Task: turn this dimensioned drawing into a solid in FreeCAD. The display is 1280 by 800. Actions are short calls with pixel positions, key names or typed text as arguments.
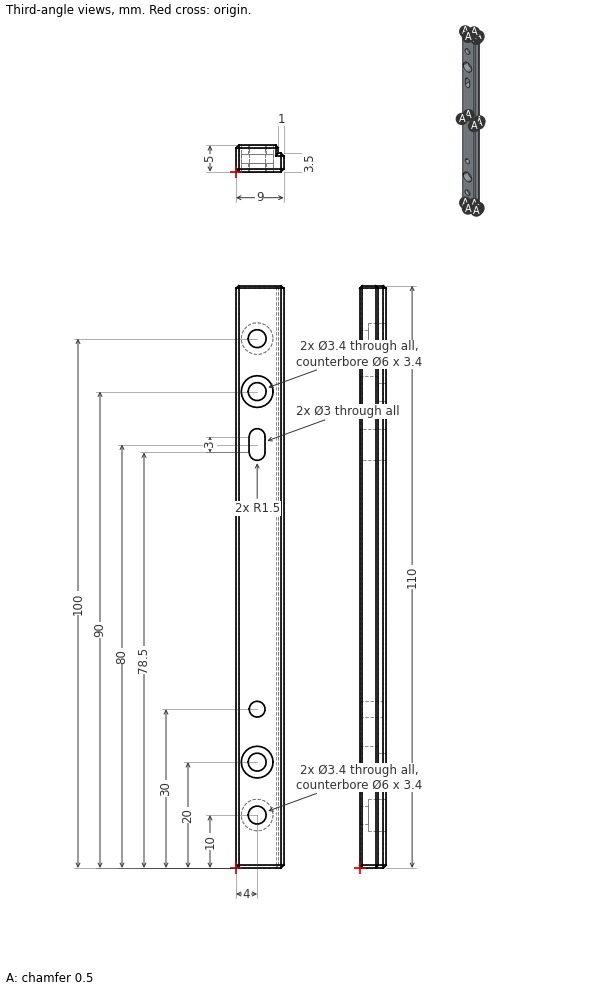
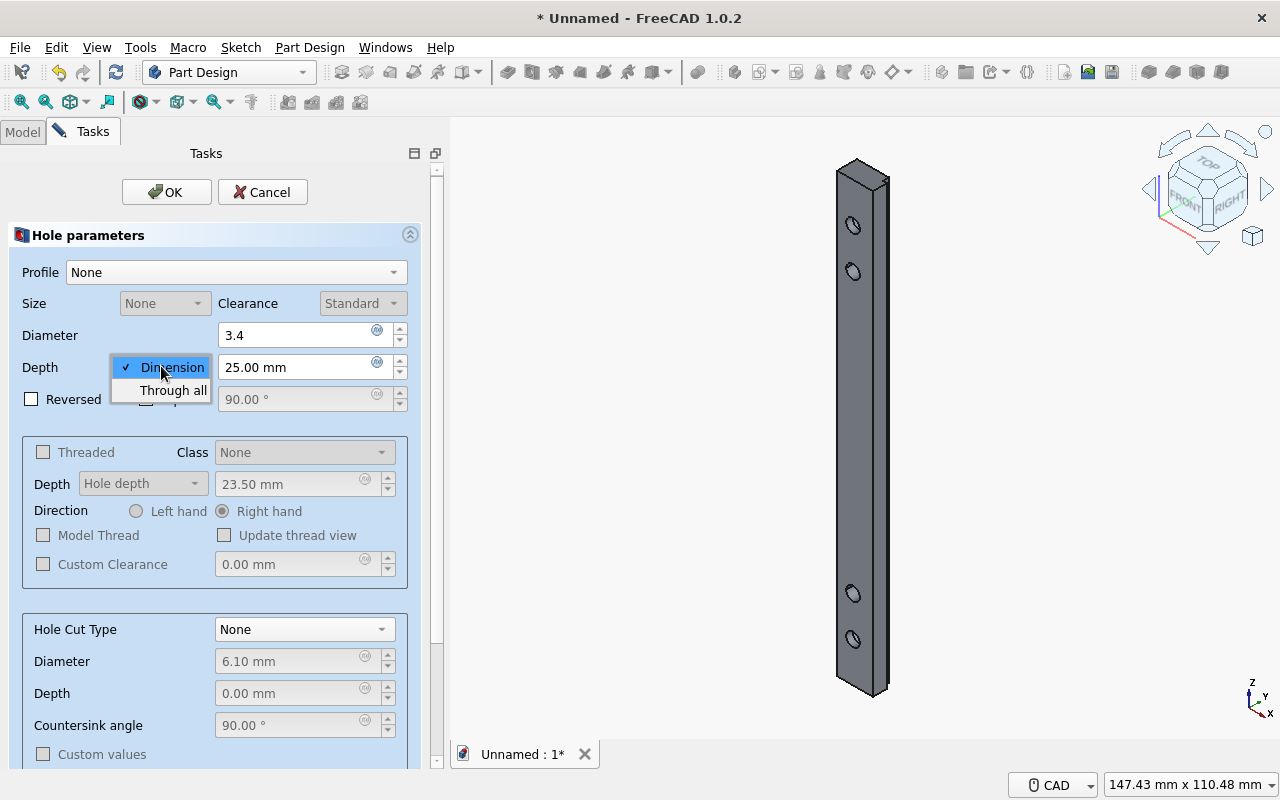
click(160, 390)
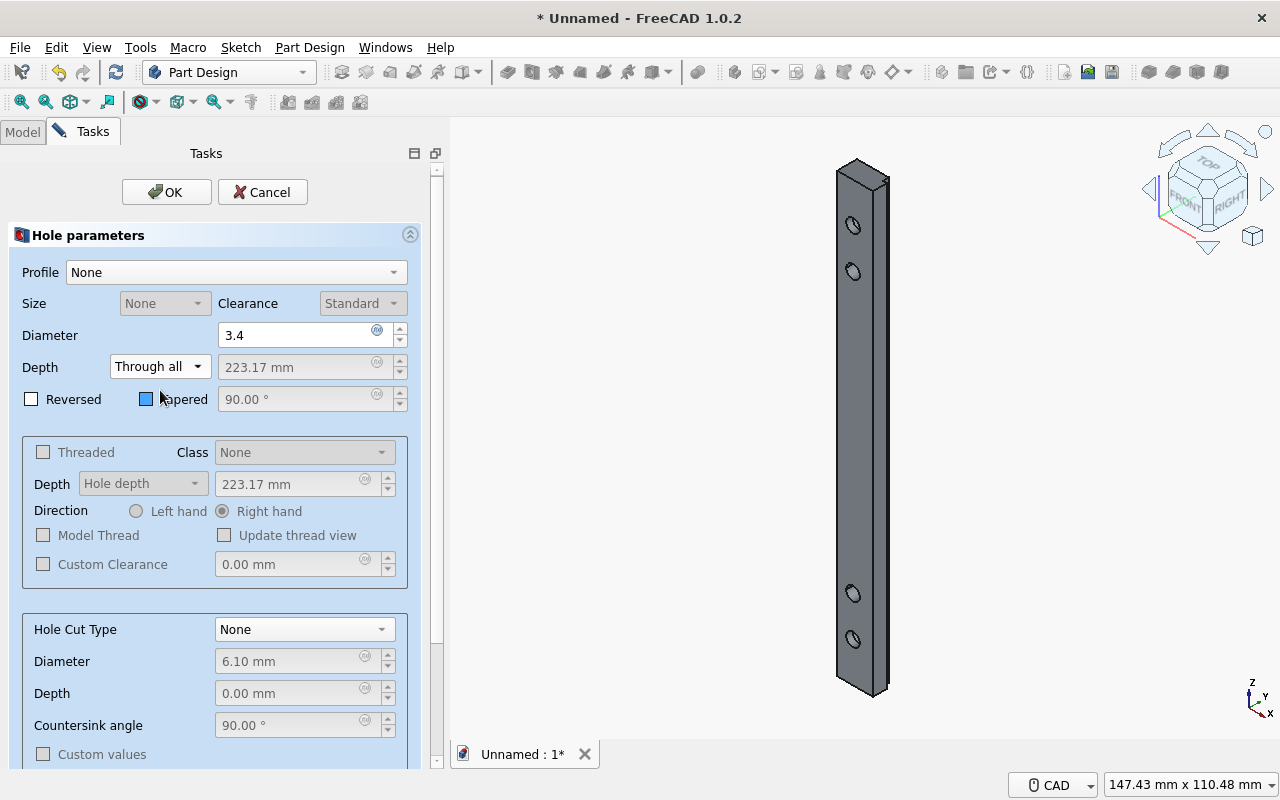
click(306, 630)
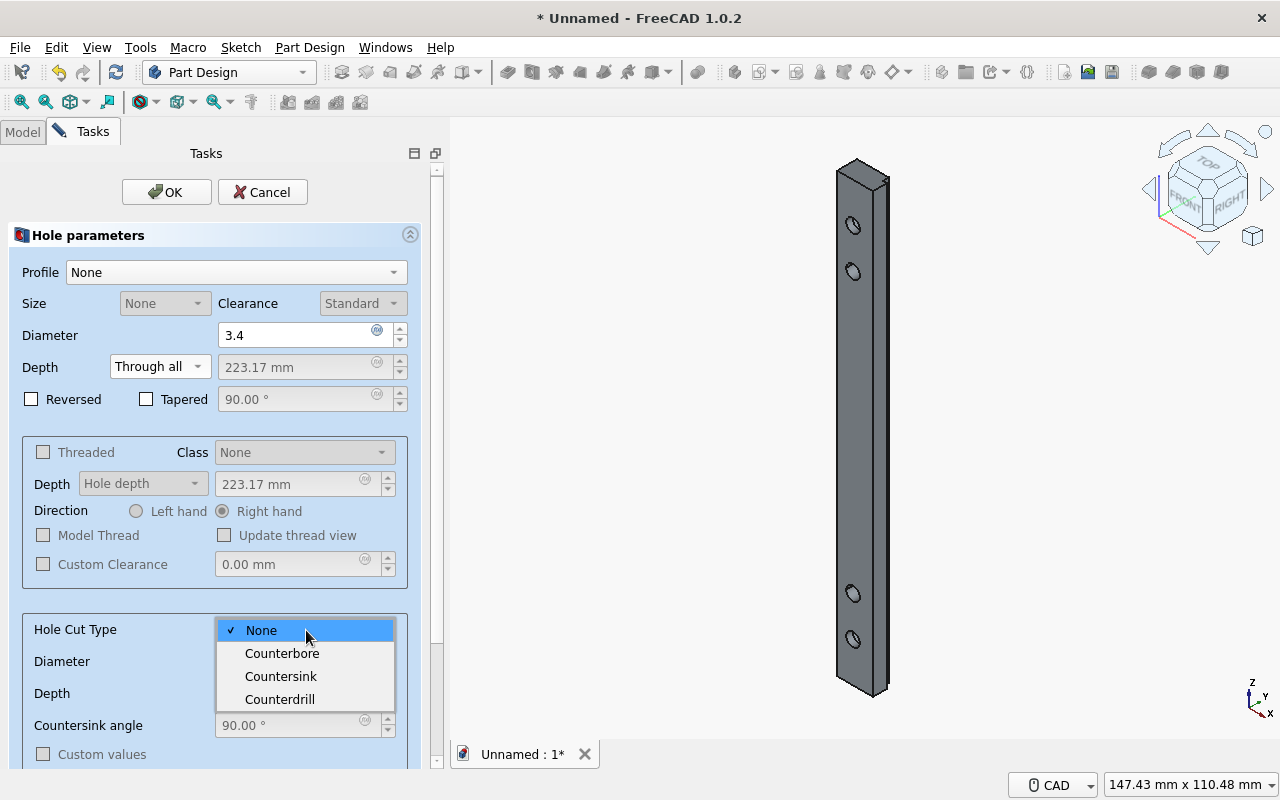
click(304, 654)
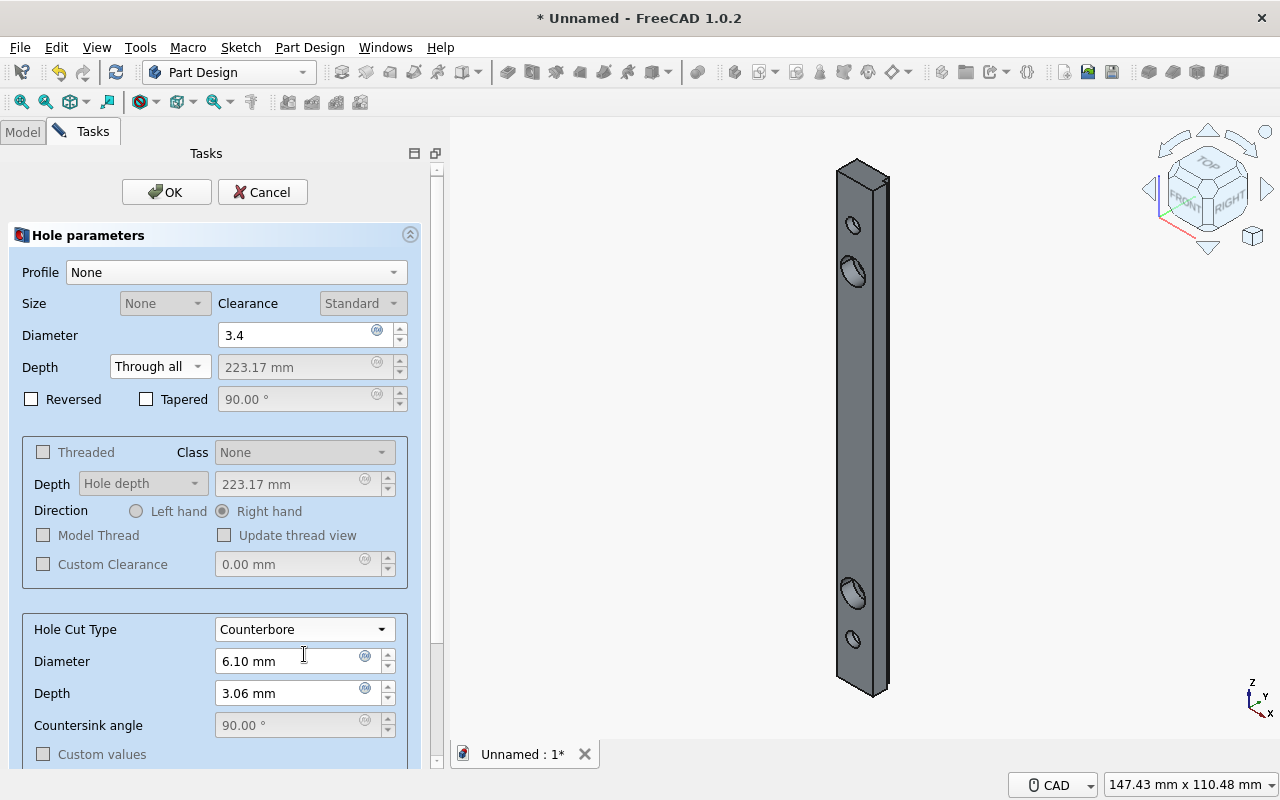
triple_click(298, 661)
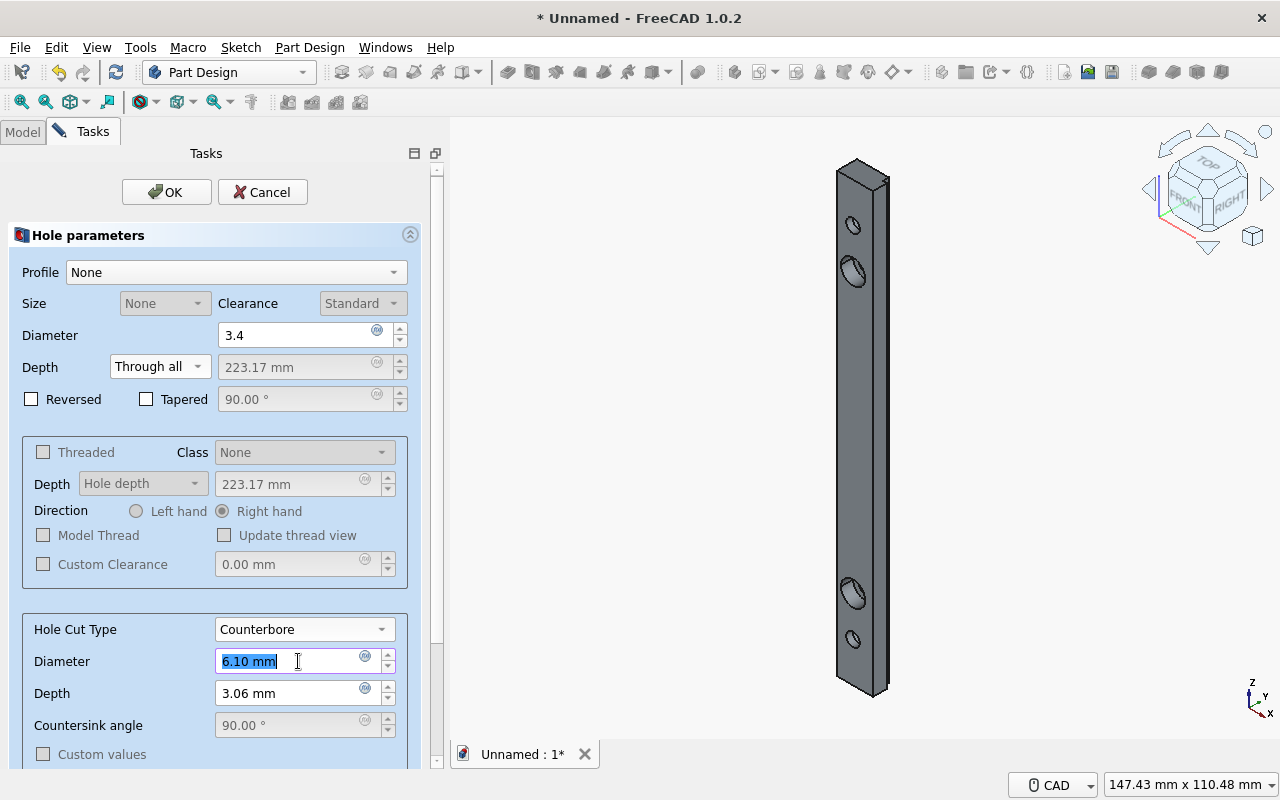
text(6)
key(Tab)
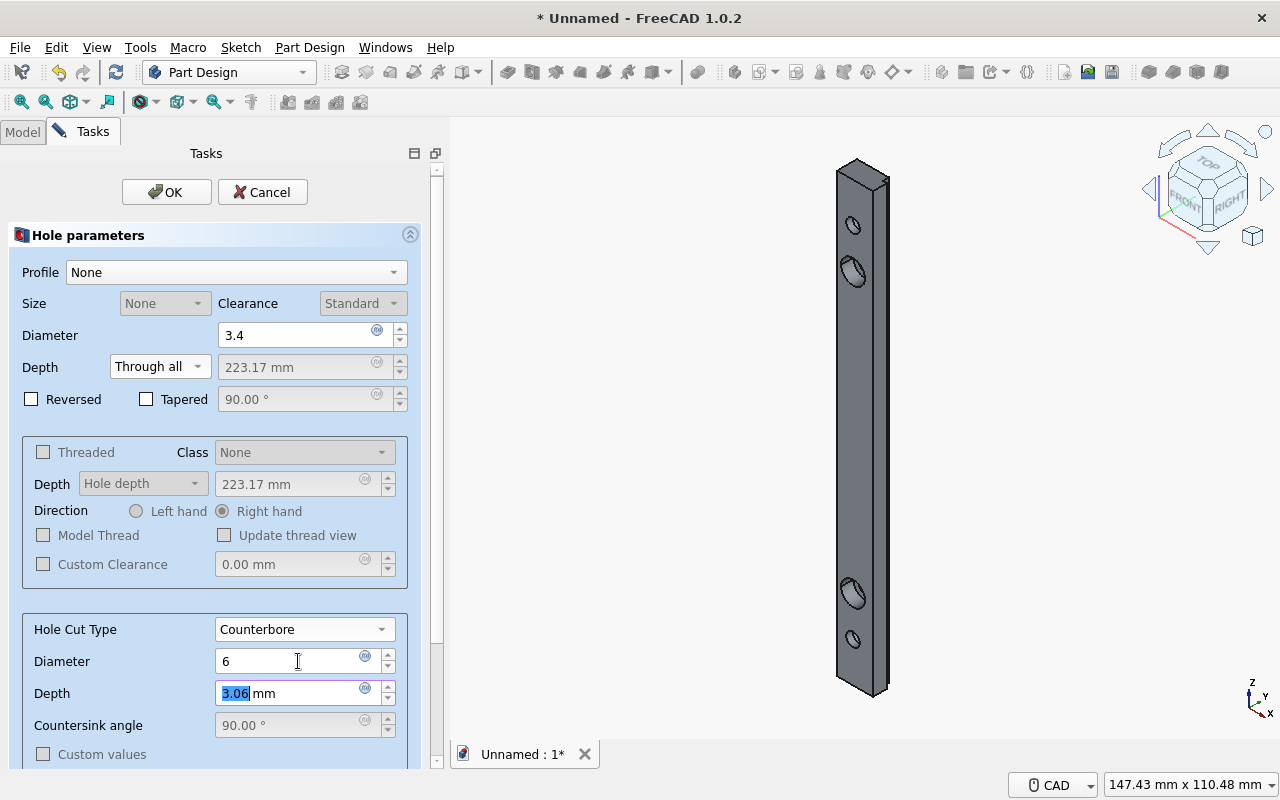
text(3.4)
key(Tab)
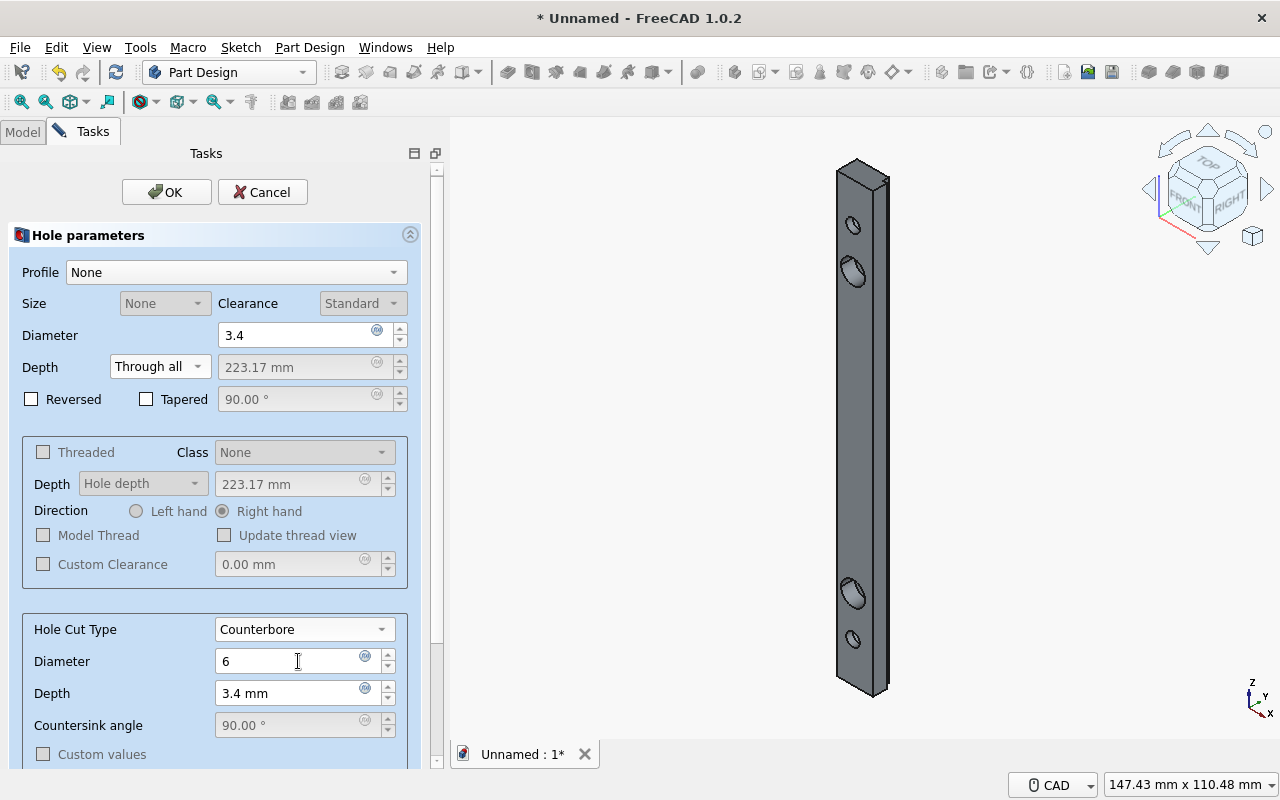
click(167, 192)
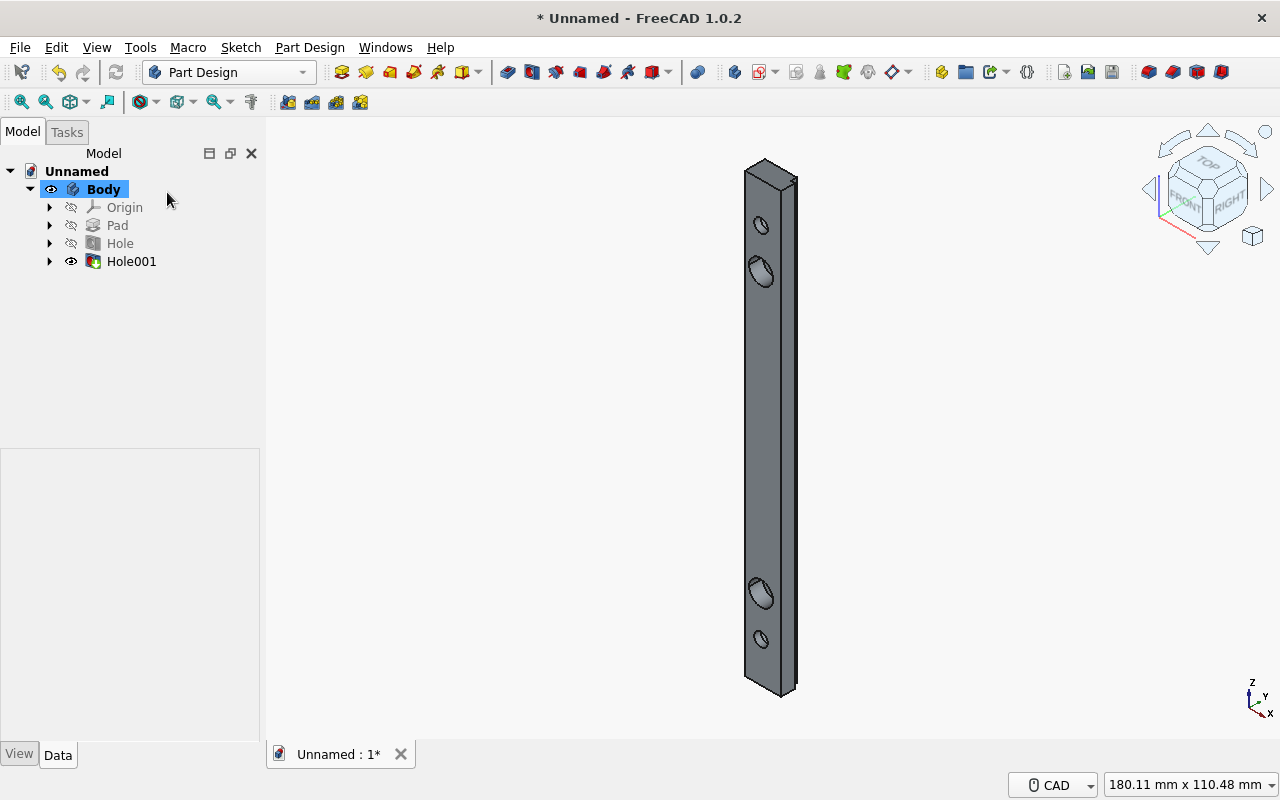
click(760, 72)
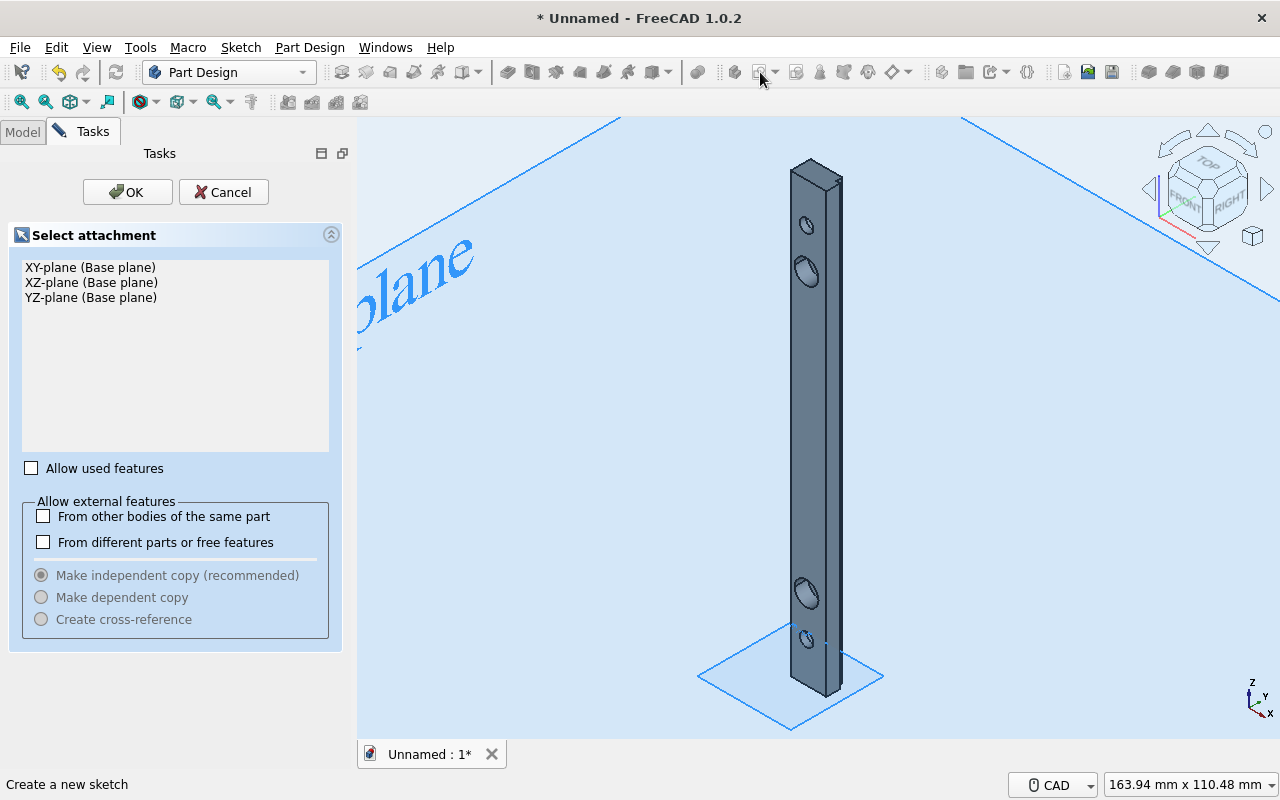
click(82, 282)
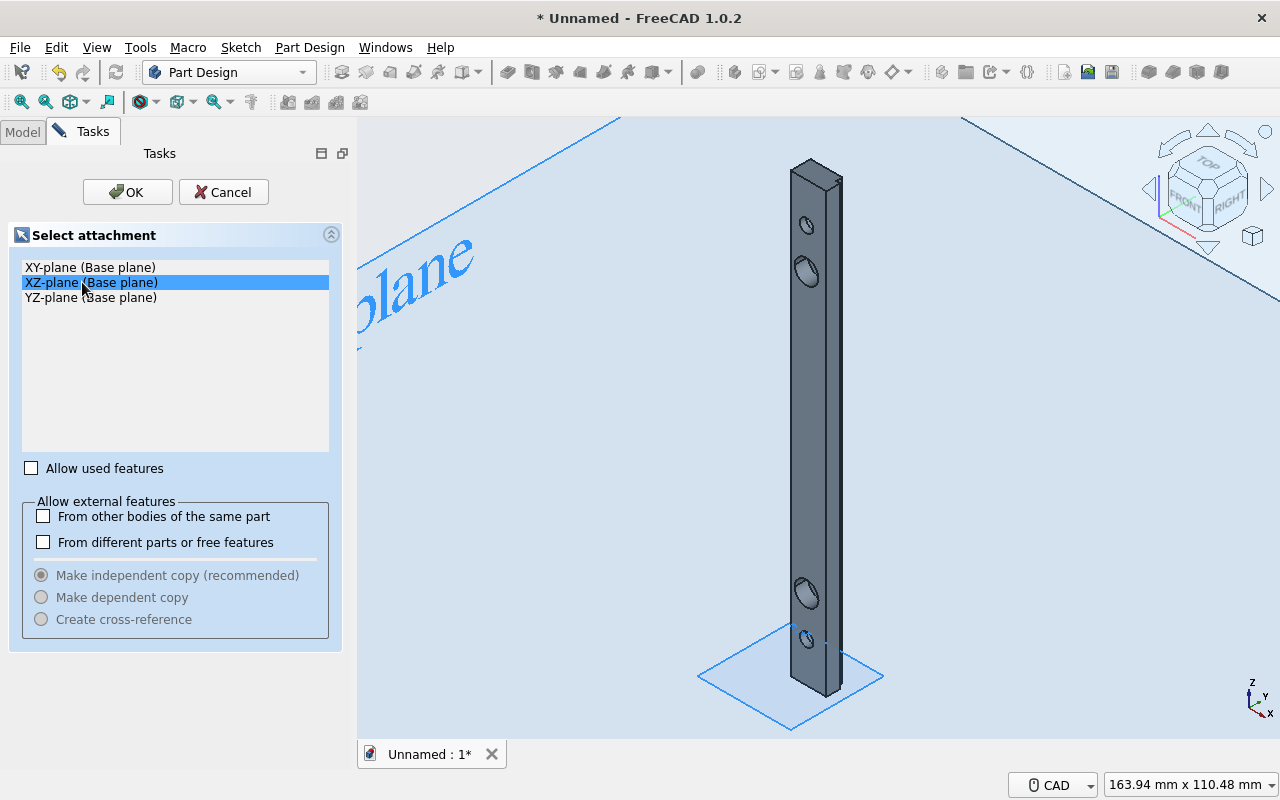
click(128, 192)